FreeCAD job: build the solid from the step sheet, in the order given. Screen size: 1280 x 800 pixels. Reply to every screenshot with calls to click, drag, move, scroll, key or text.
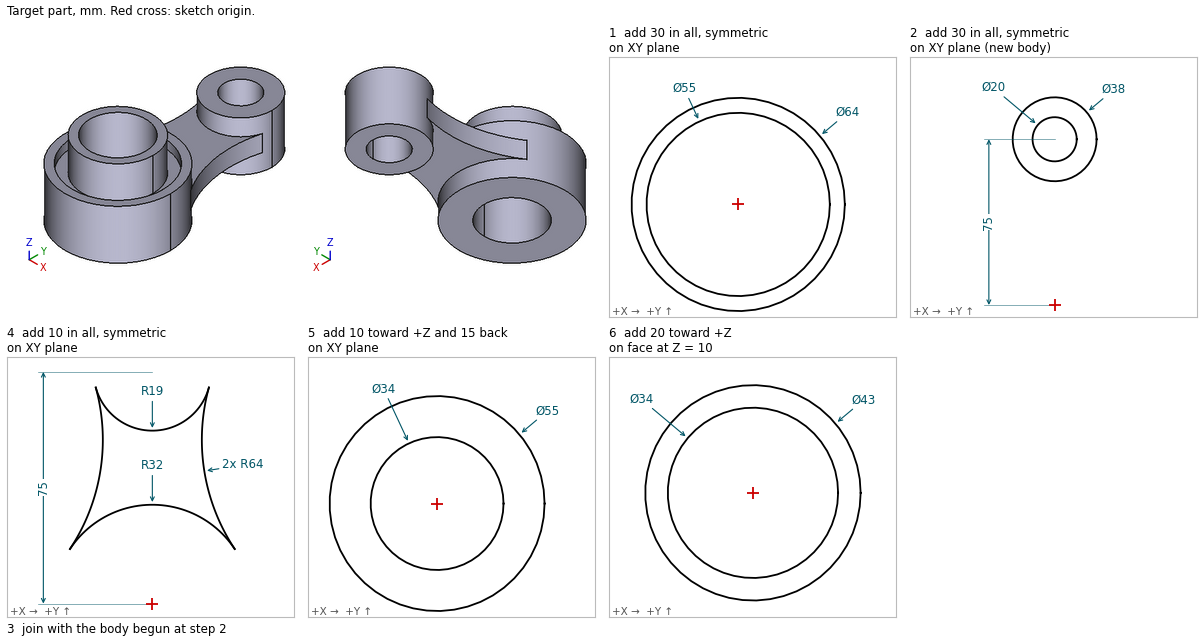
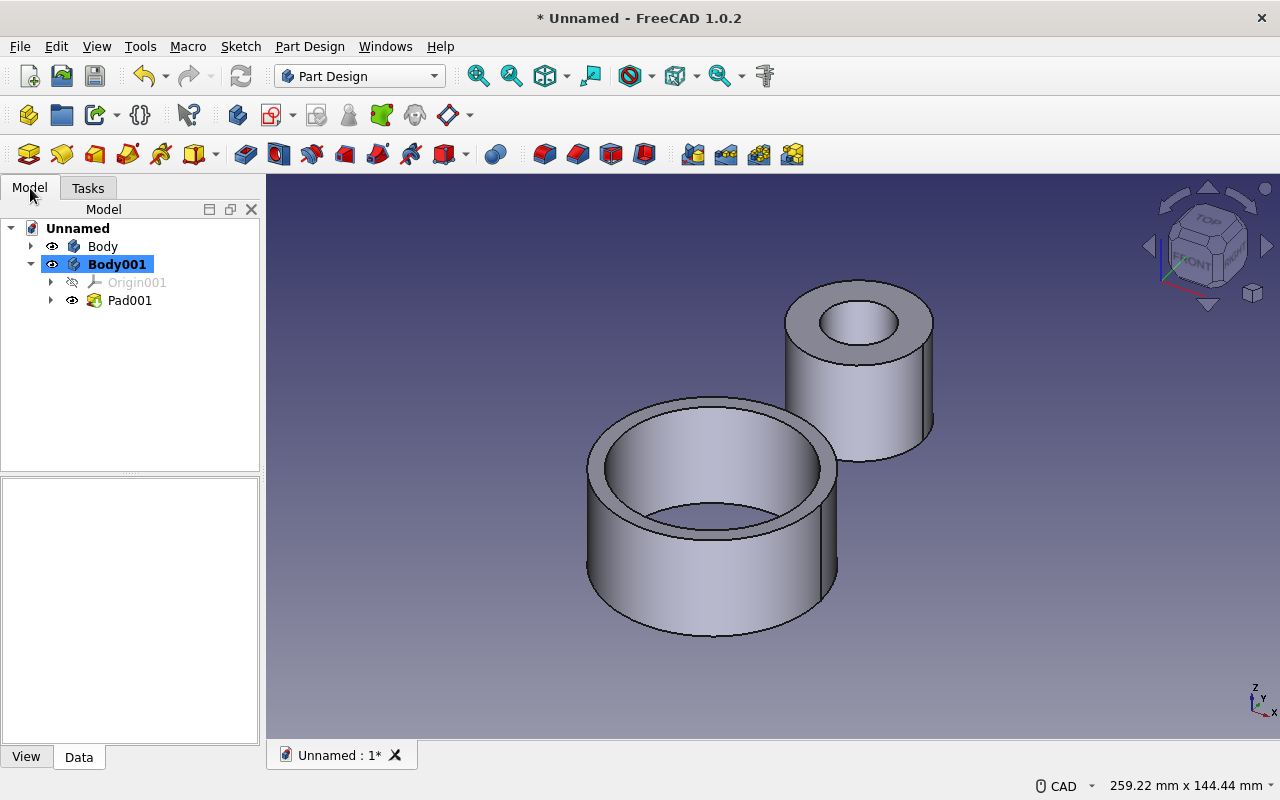
double_click(97, 246)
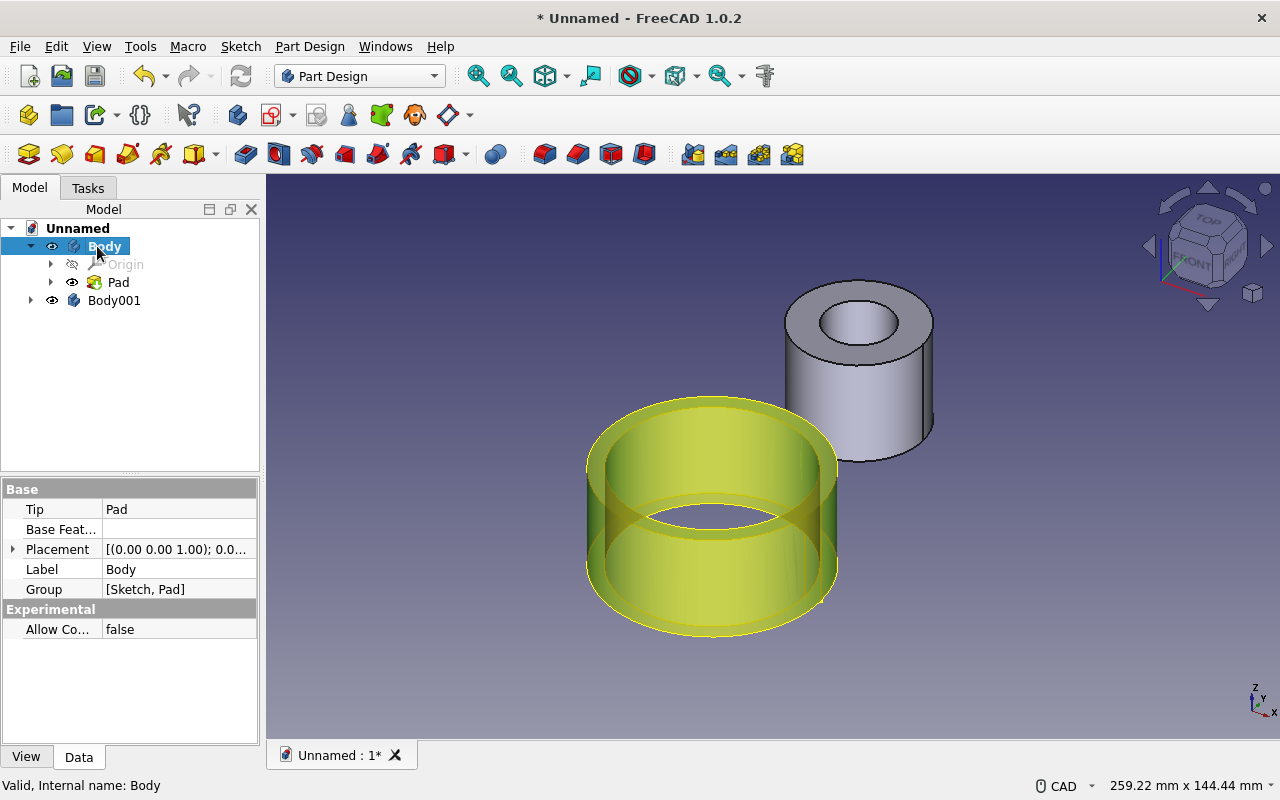
click(97, 246)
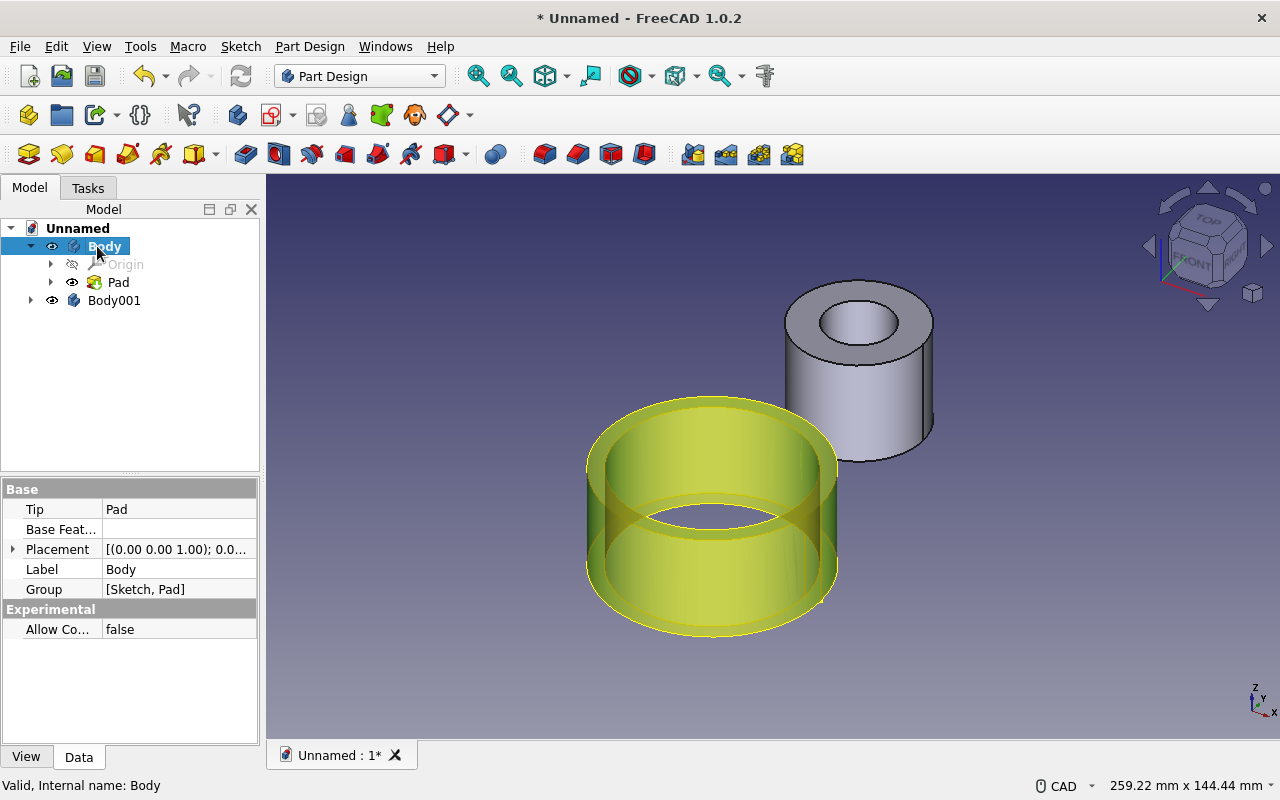
click(148, 629)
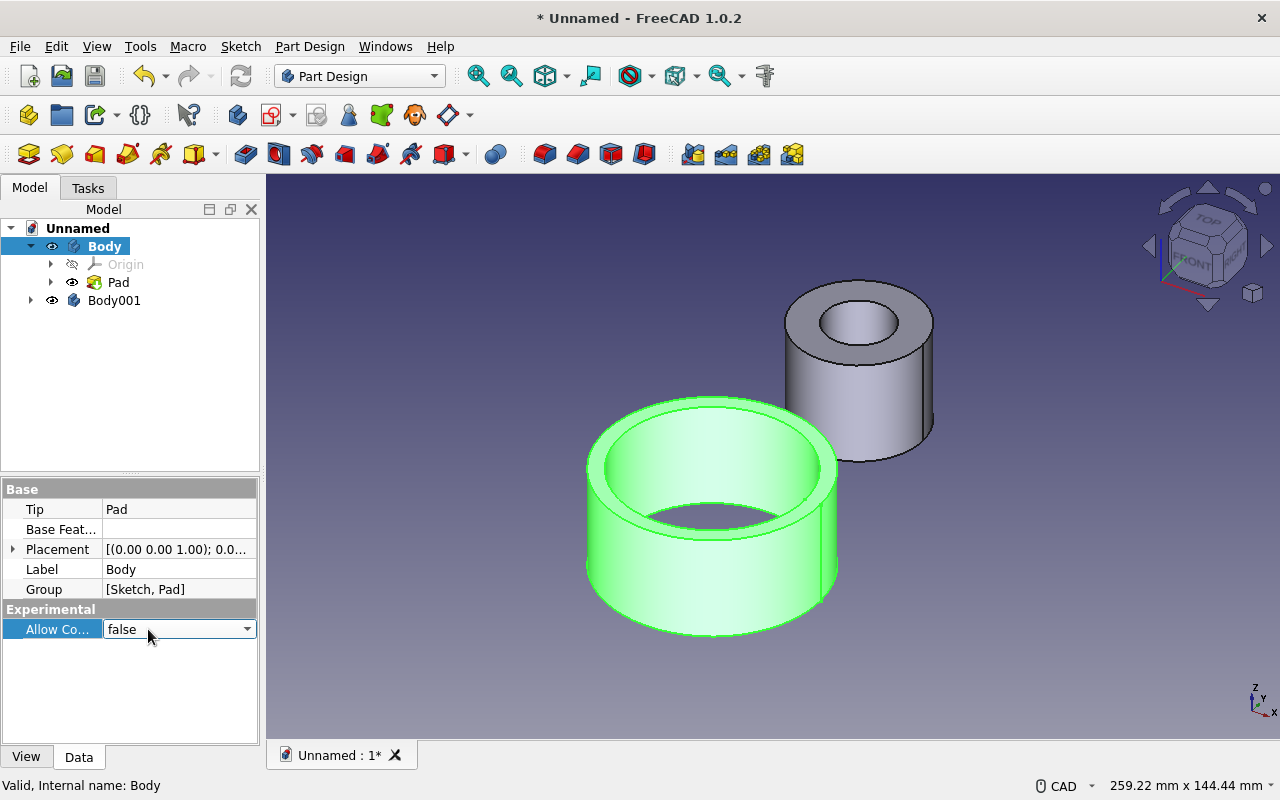
click(148, 629)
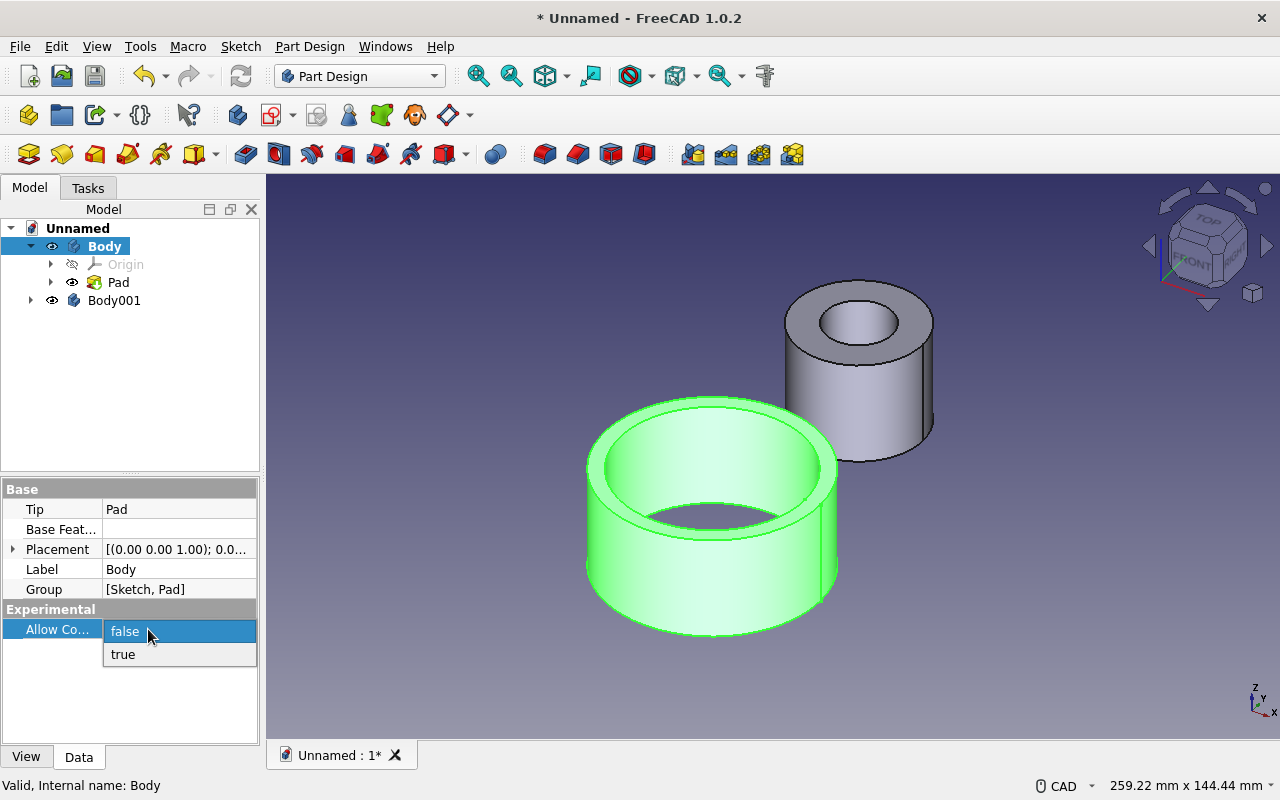
click(178, 654)
key(Return)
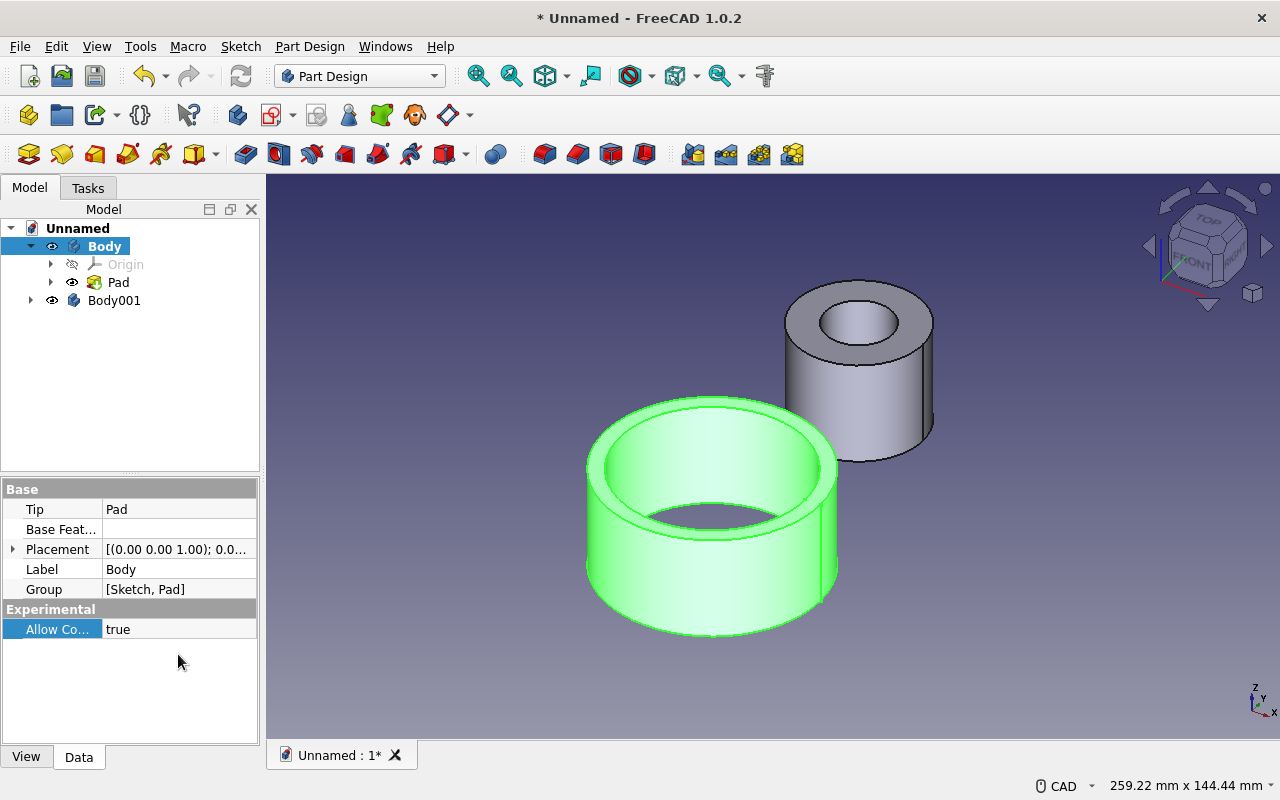
click(97, 300)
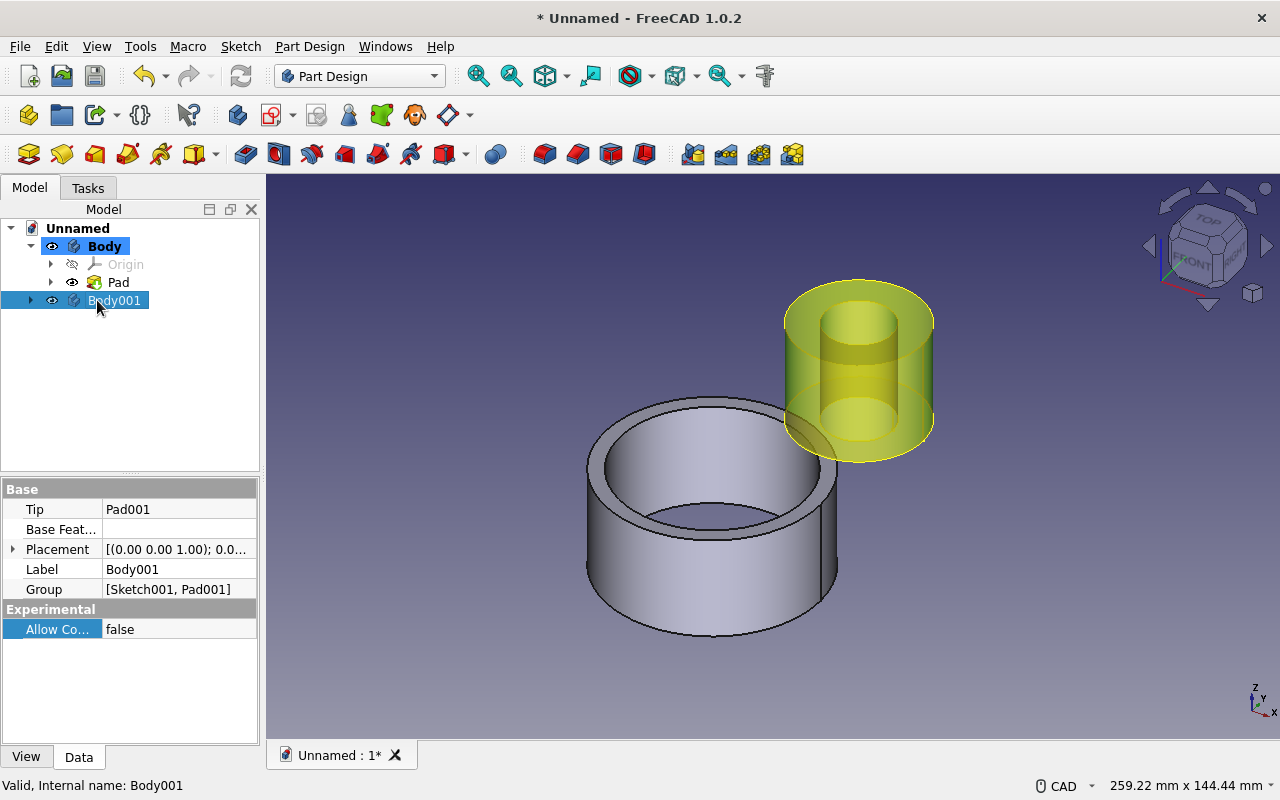
click(496, 154)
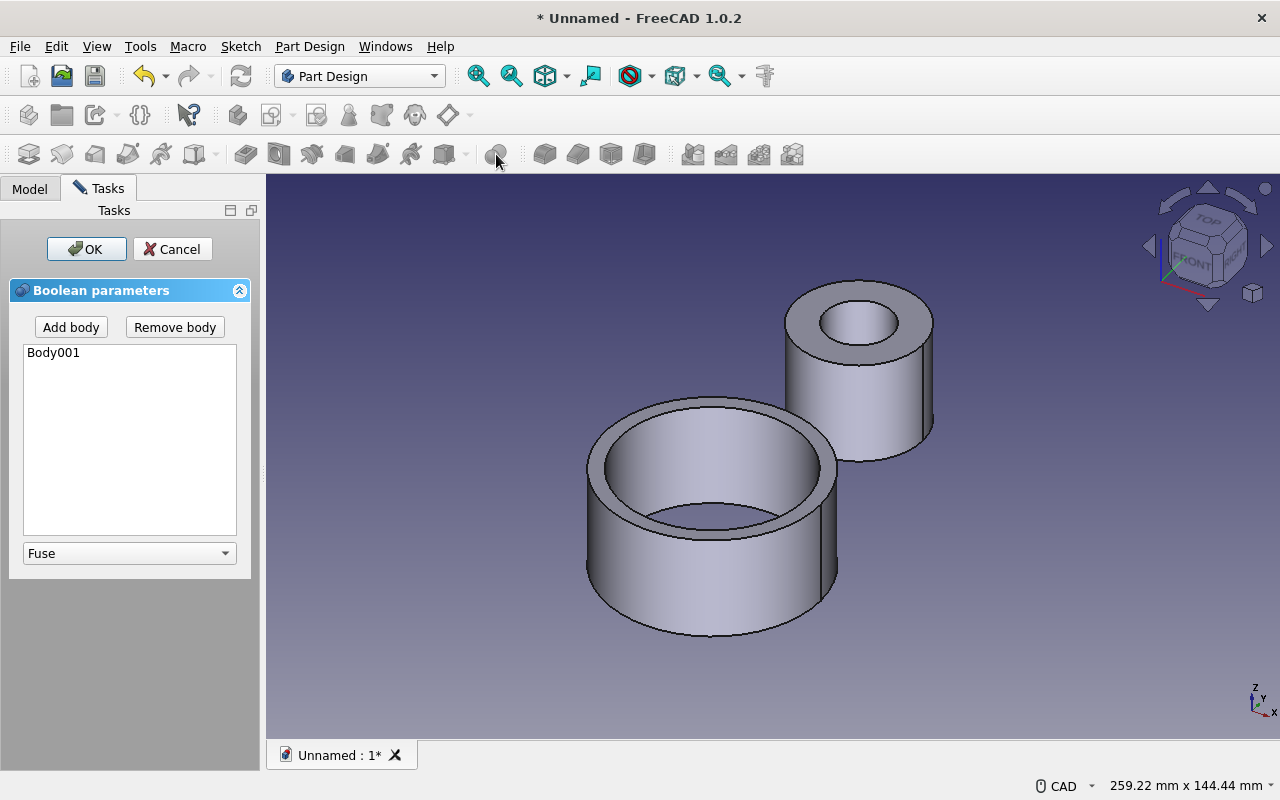
click(87, 249)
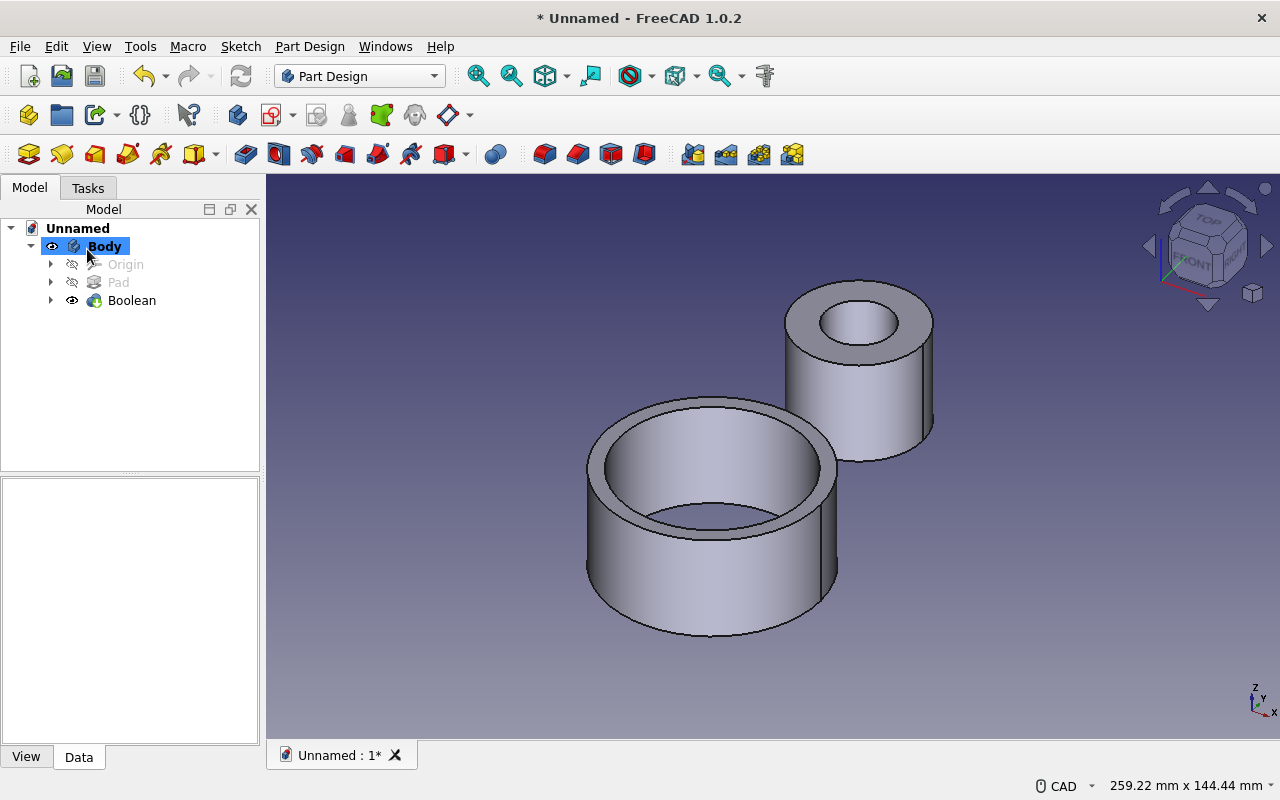
click(270, 116)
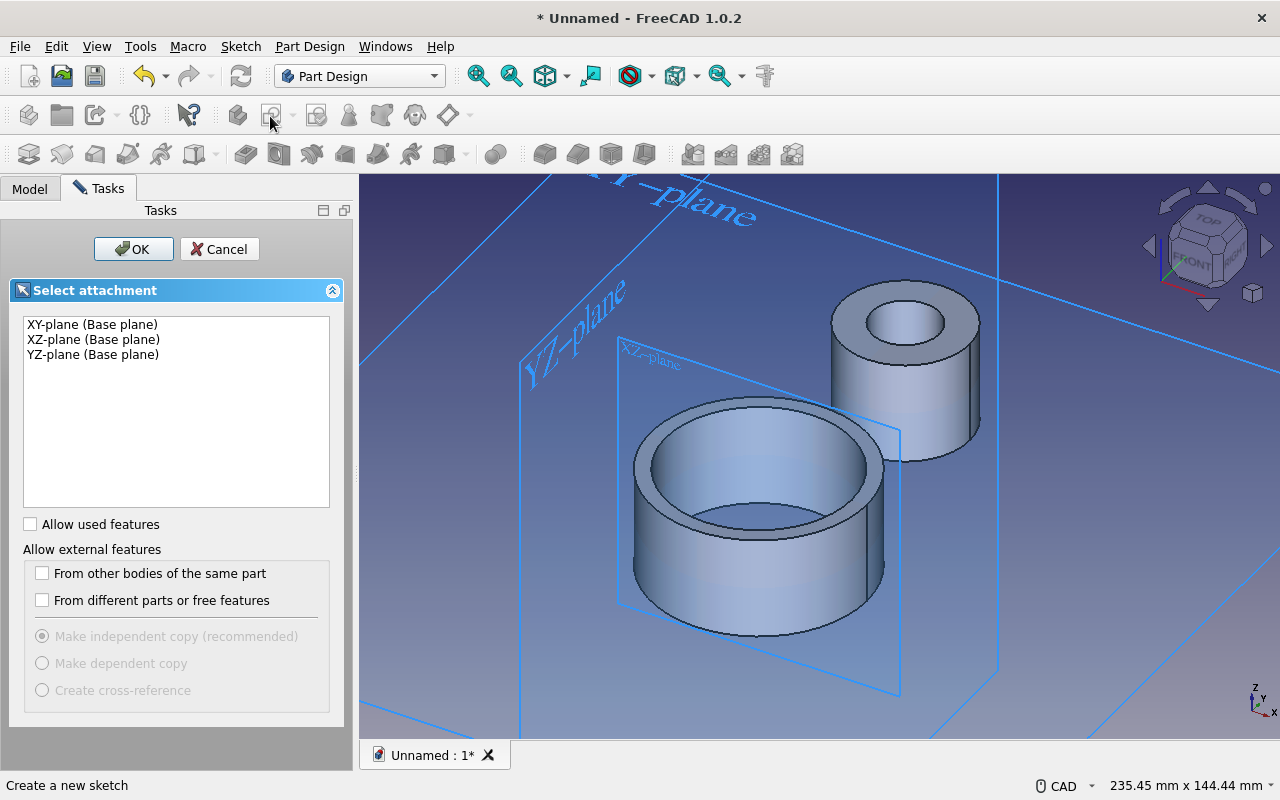
click(84, 324)